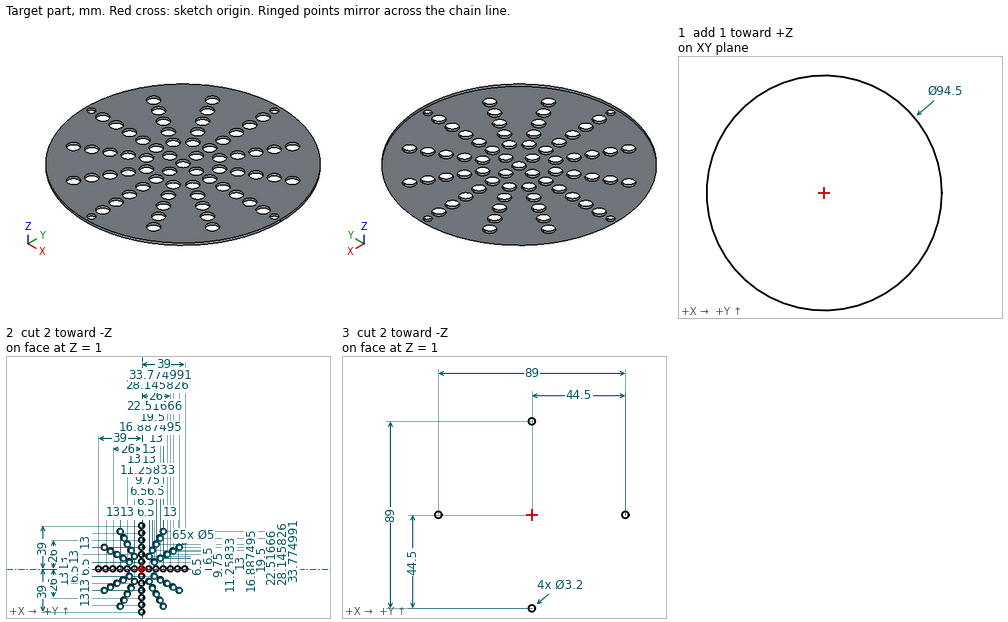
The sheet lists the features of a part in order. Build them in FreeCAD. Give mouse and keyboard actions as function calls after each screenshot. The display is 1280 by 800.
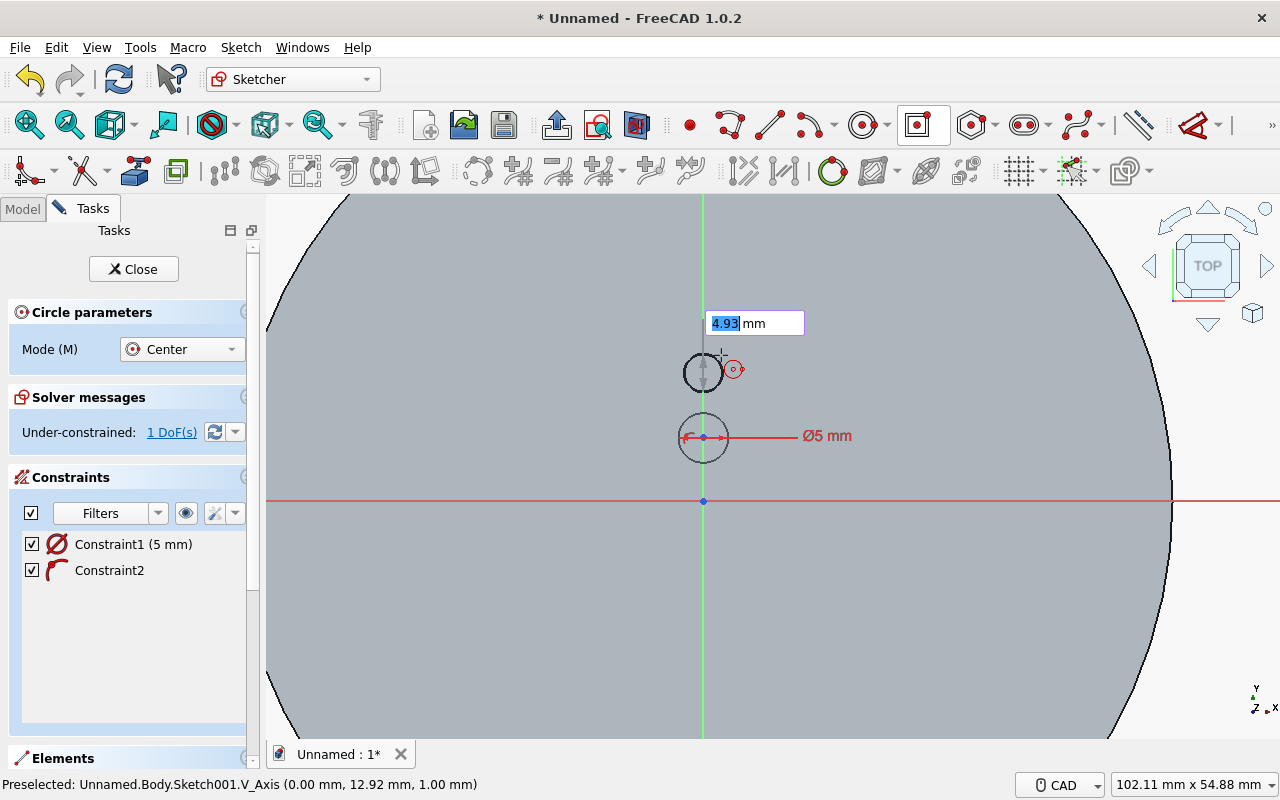
text(5)
key(Return)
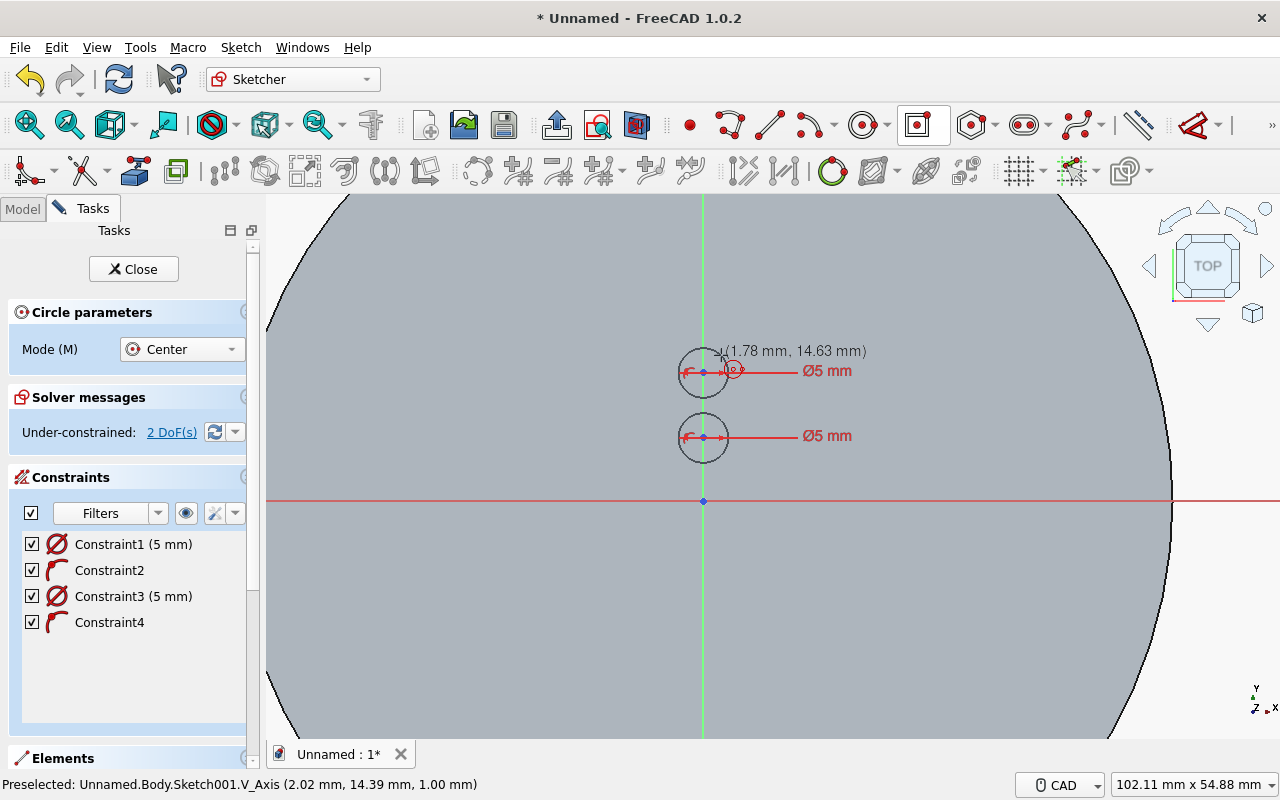
click(703, 308)
move(721, 290)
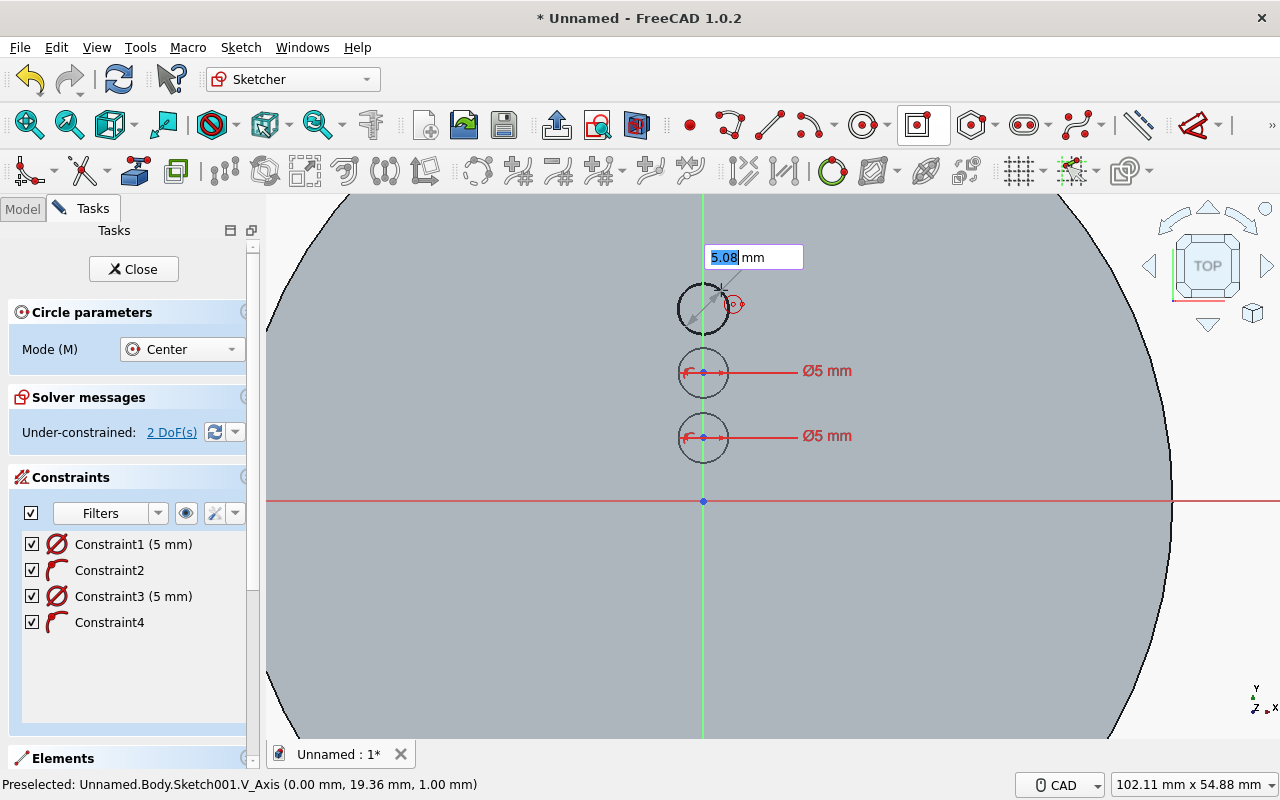
text(5)
key(Return)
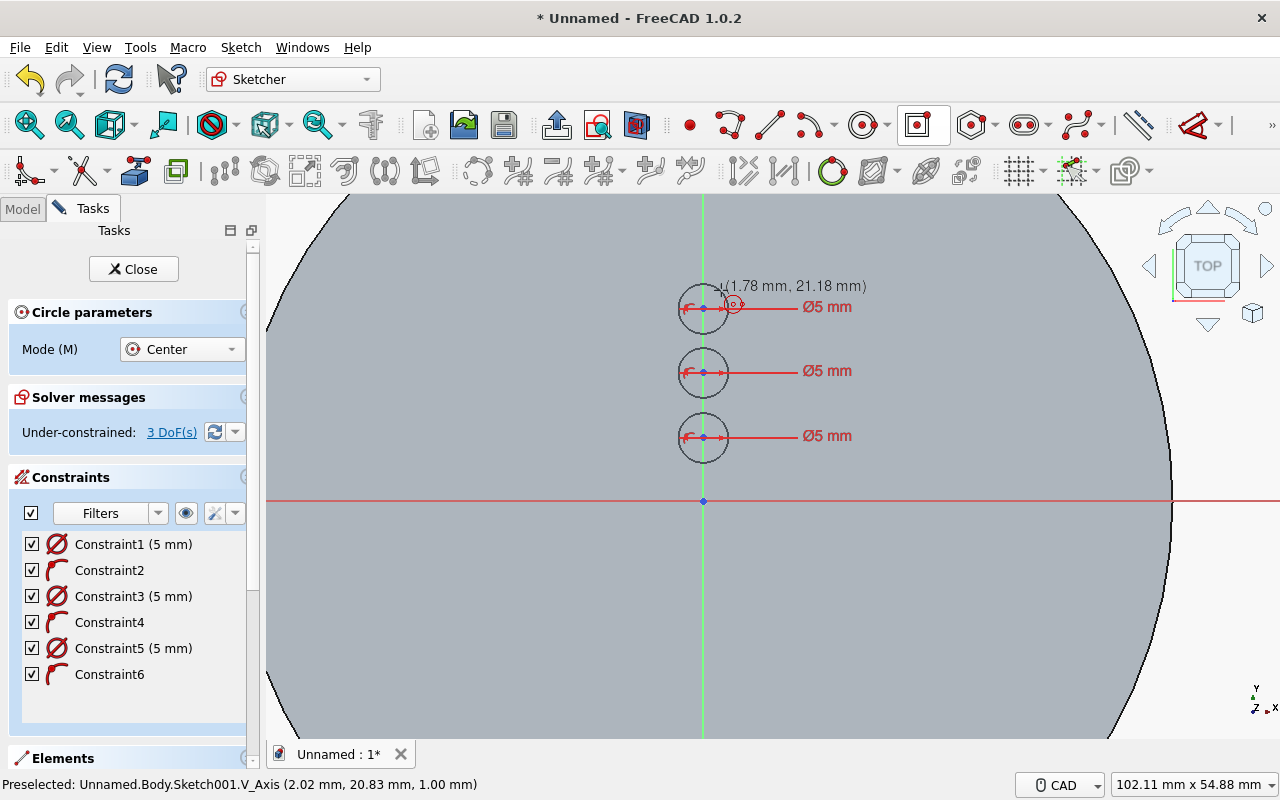
click(703, 243)
move(721, 226)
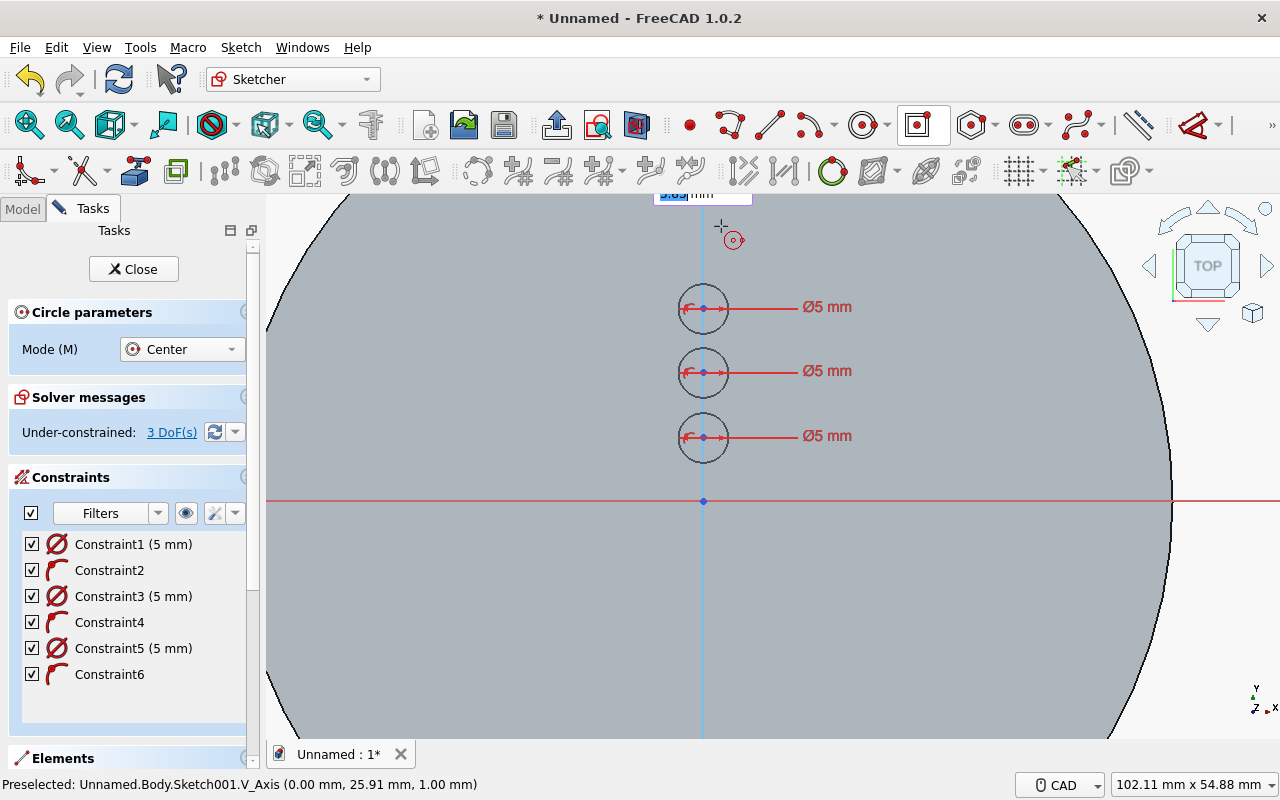
text(5)
key(Return)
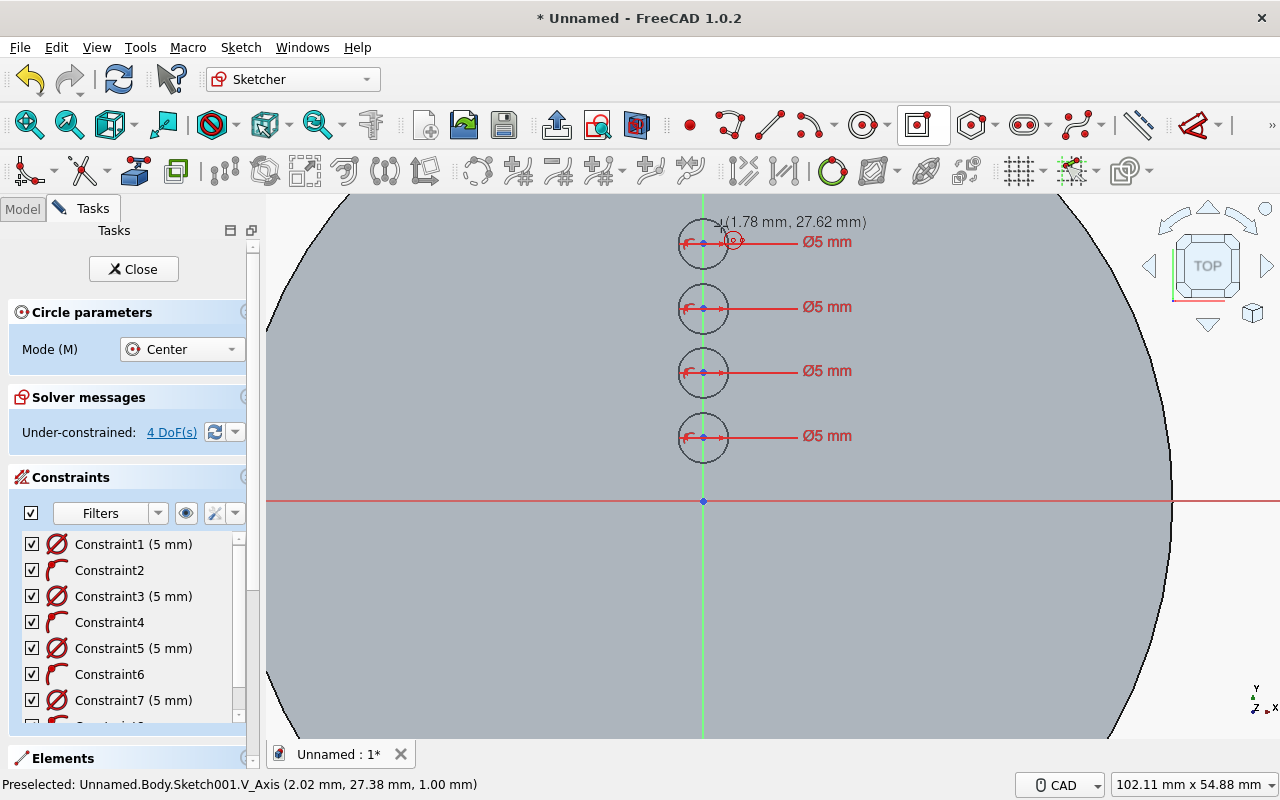
scroll(705, 438, down, 4)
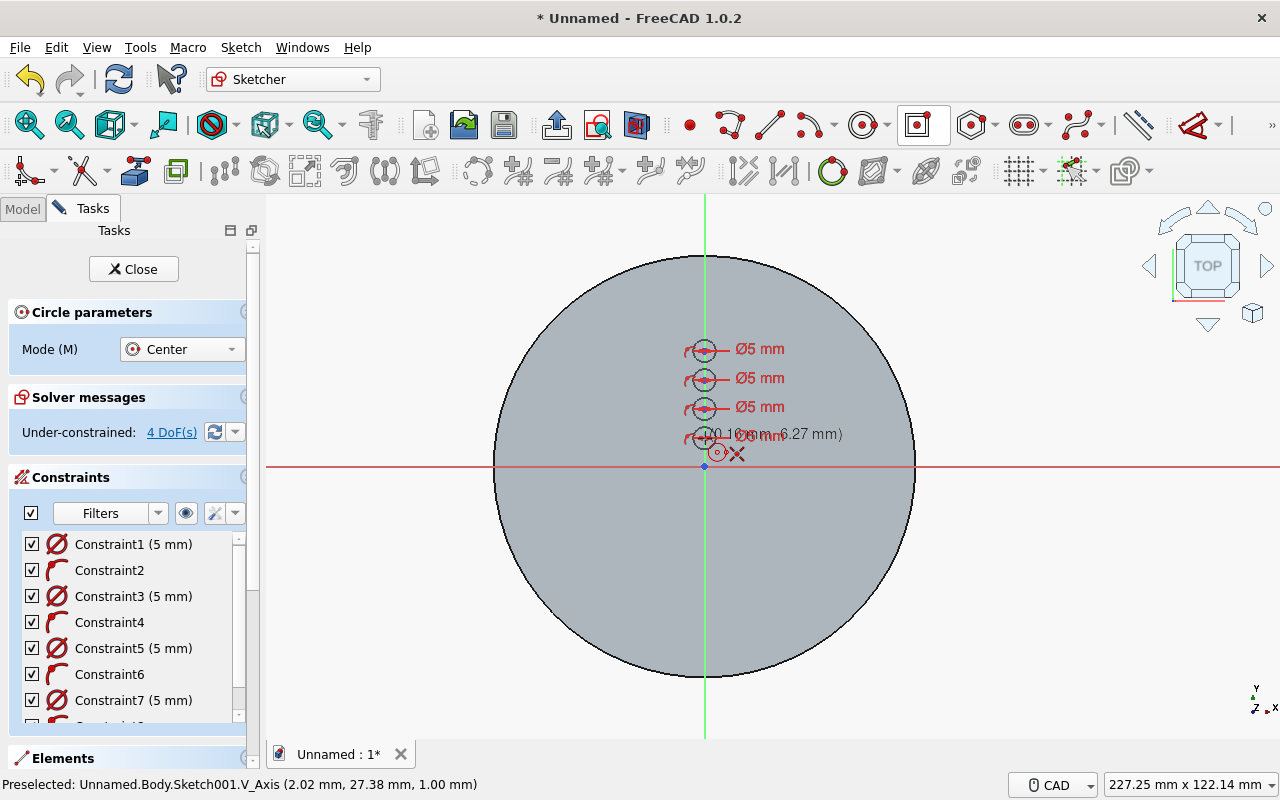
scroll(705, 322, up, 4)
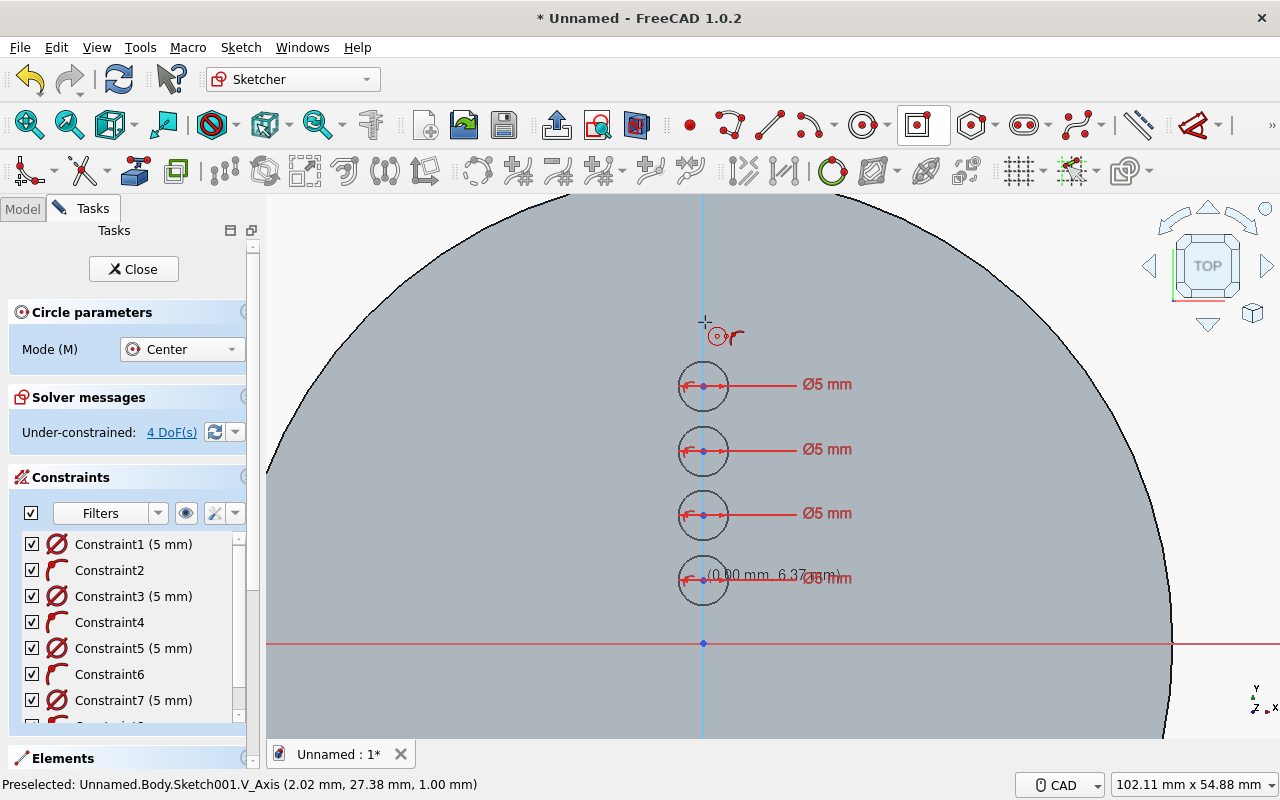
click(703, 321)
move(721, 303)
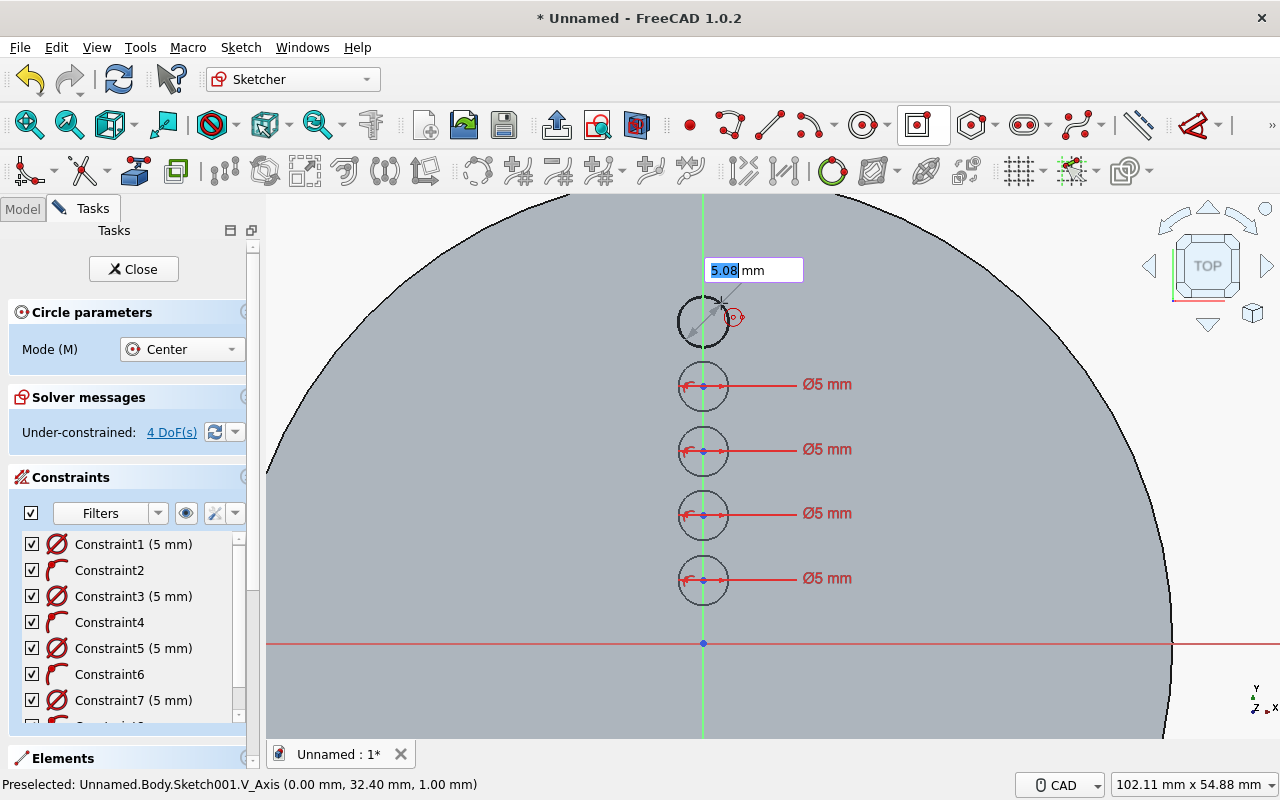
text(5)
key(Return)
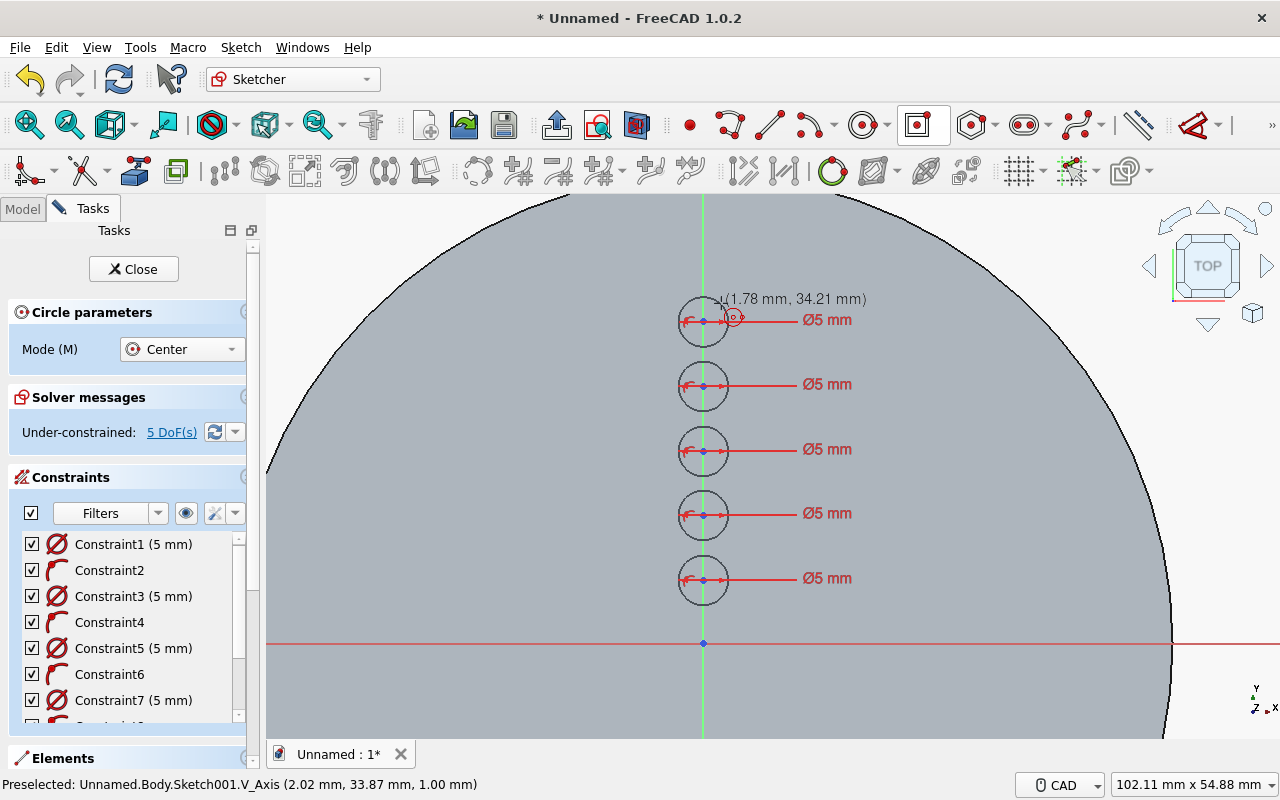
click(703, 256)
move(721, 239)